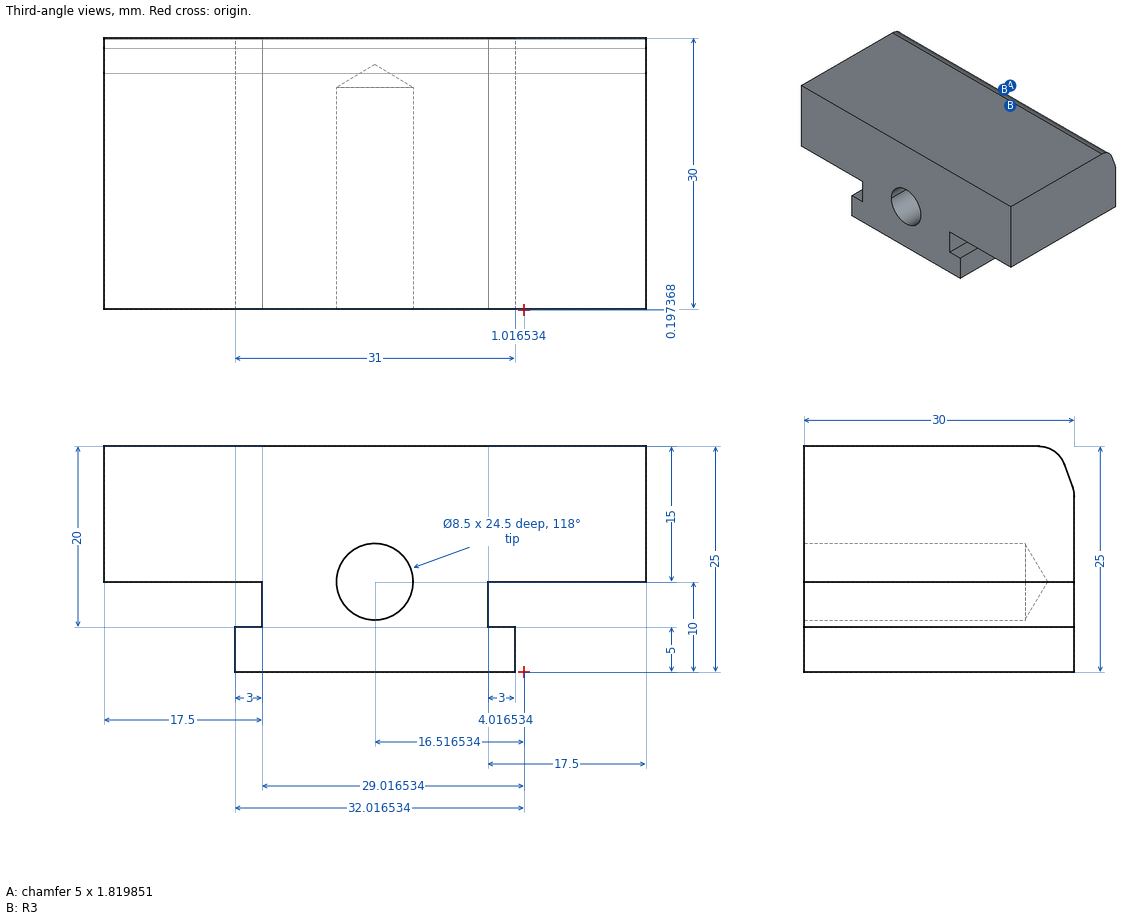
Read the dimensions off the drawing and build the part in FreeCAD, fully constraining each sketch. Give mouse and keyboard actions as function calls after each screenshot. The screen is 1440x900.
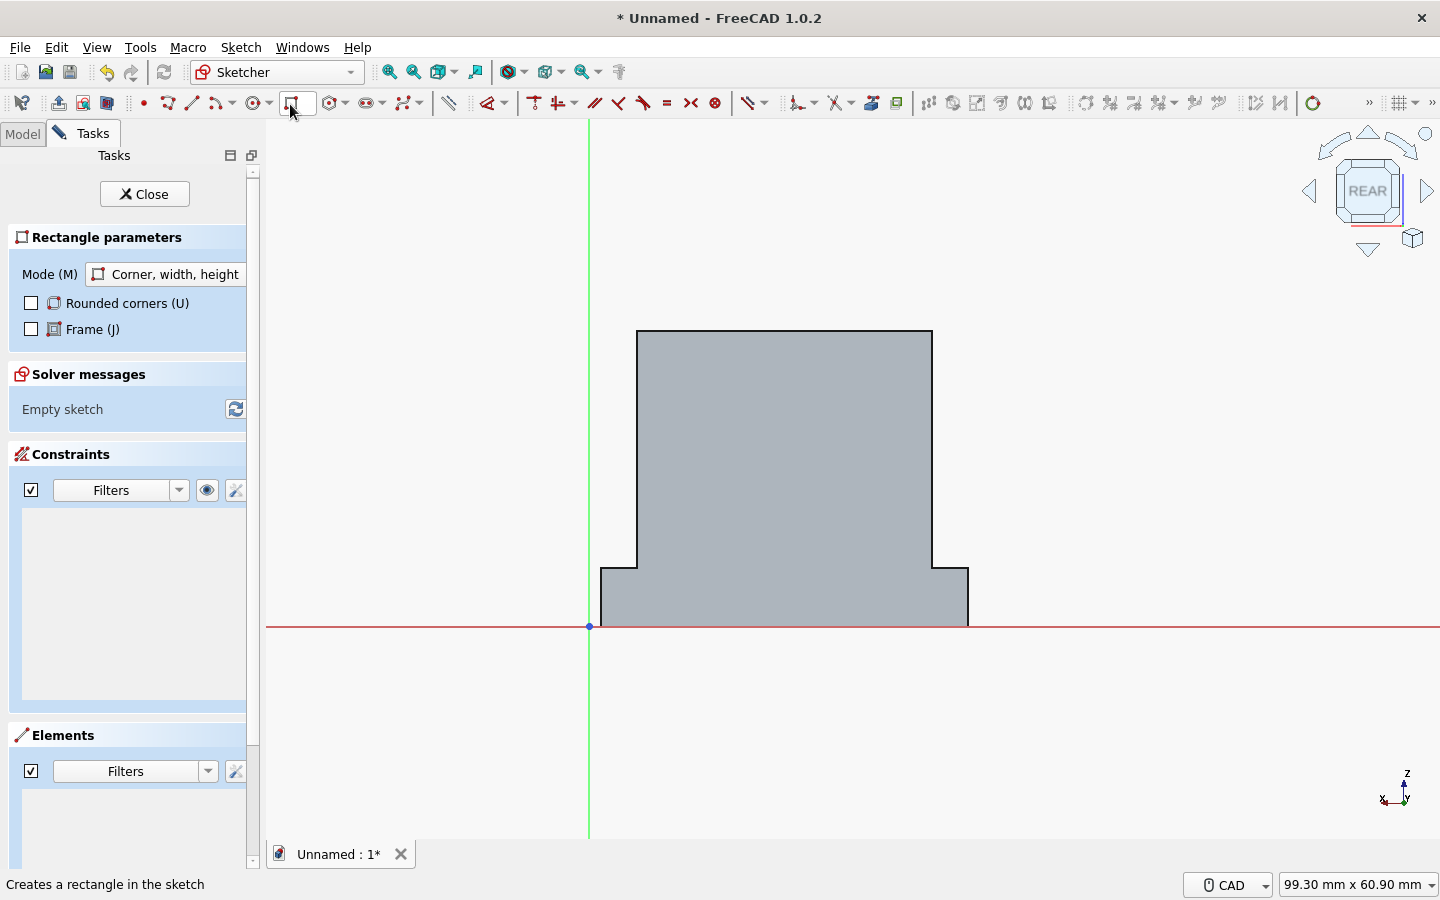
click(430, 331)
move(637, 509)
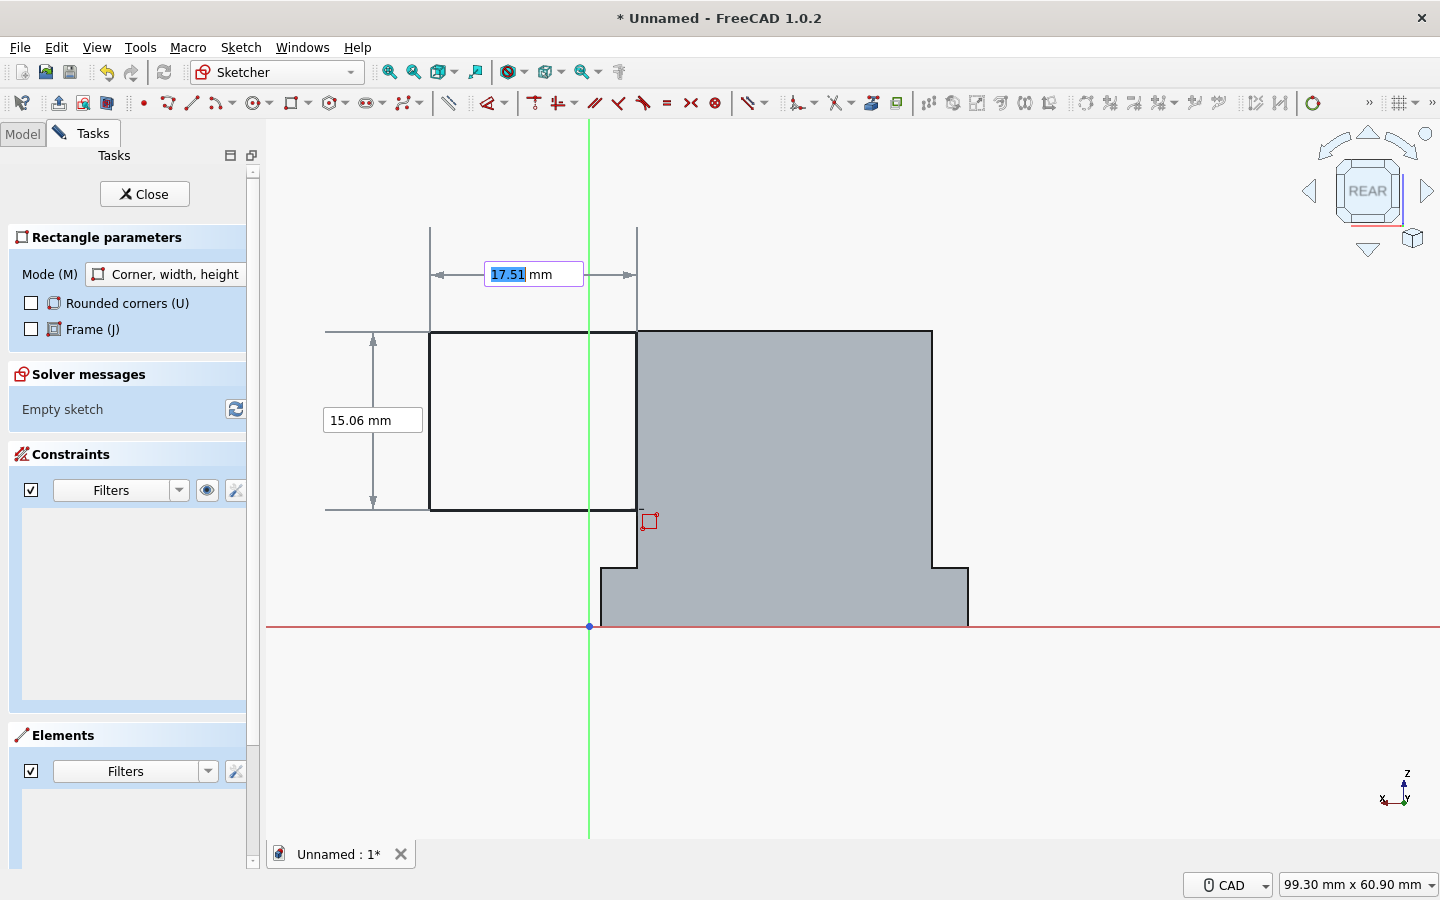
text(17.5)
key(Tab)
text(15)
key(Return)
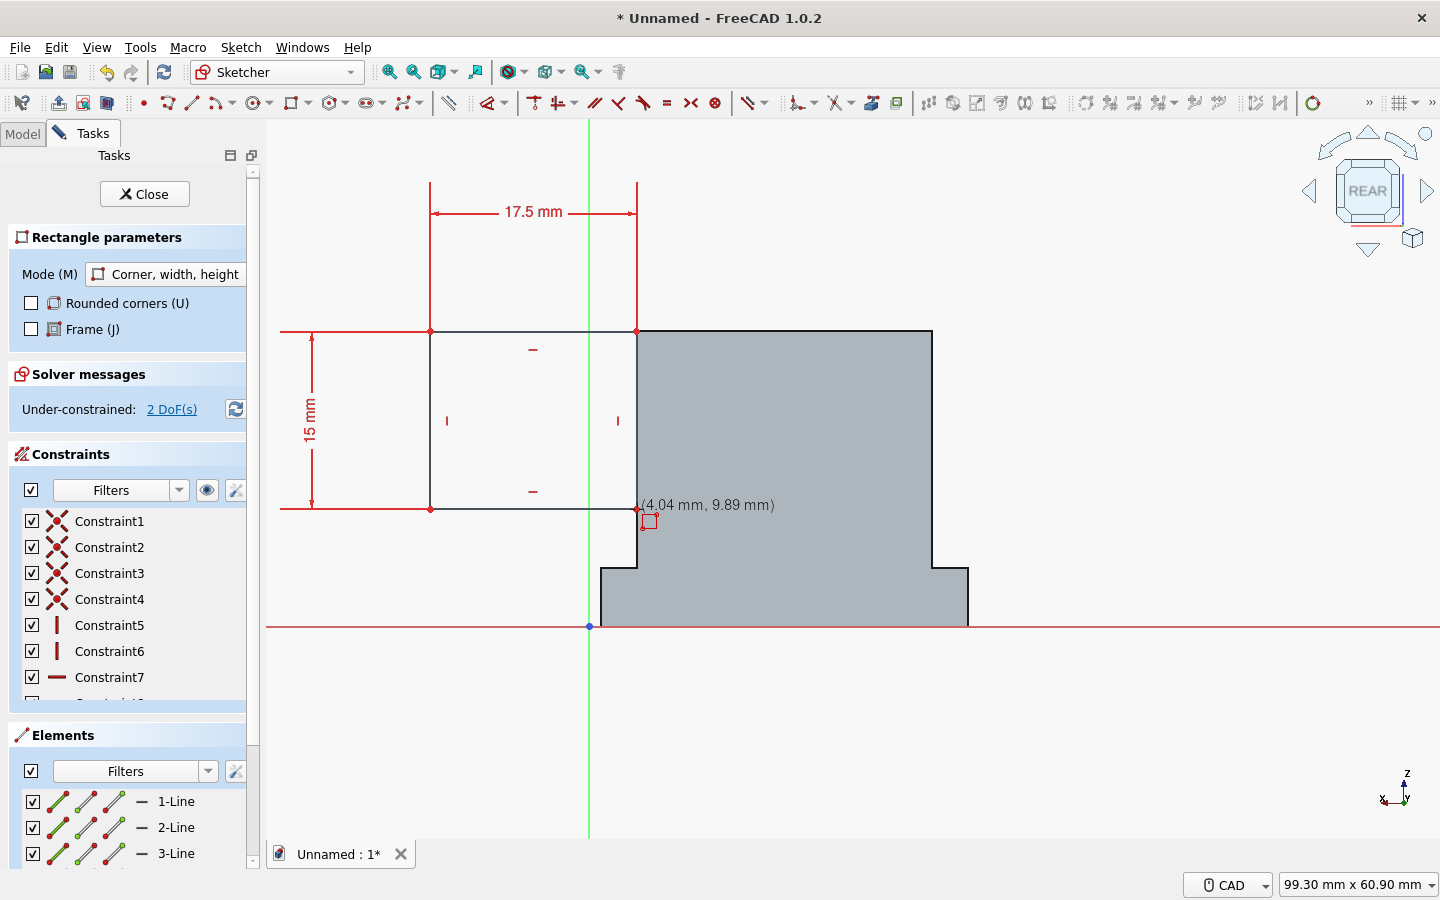
click(932, 331)
move(1139, 509)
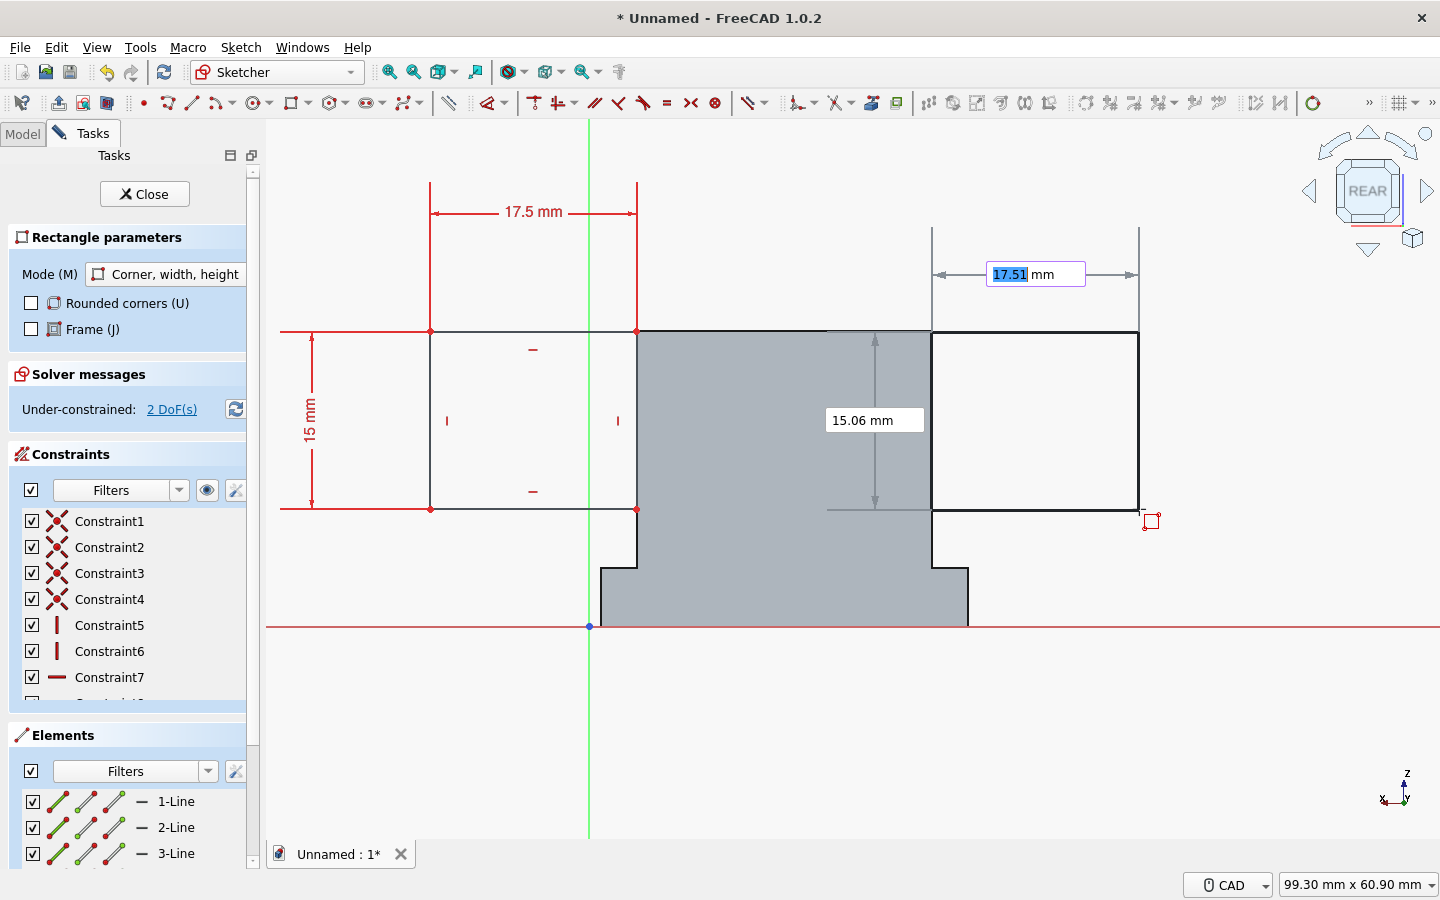
text(17.5)
key(Tab)
text(15)
key(Return)
key(Escape)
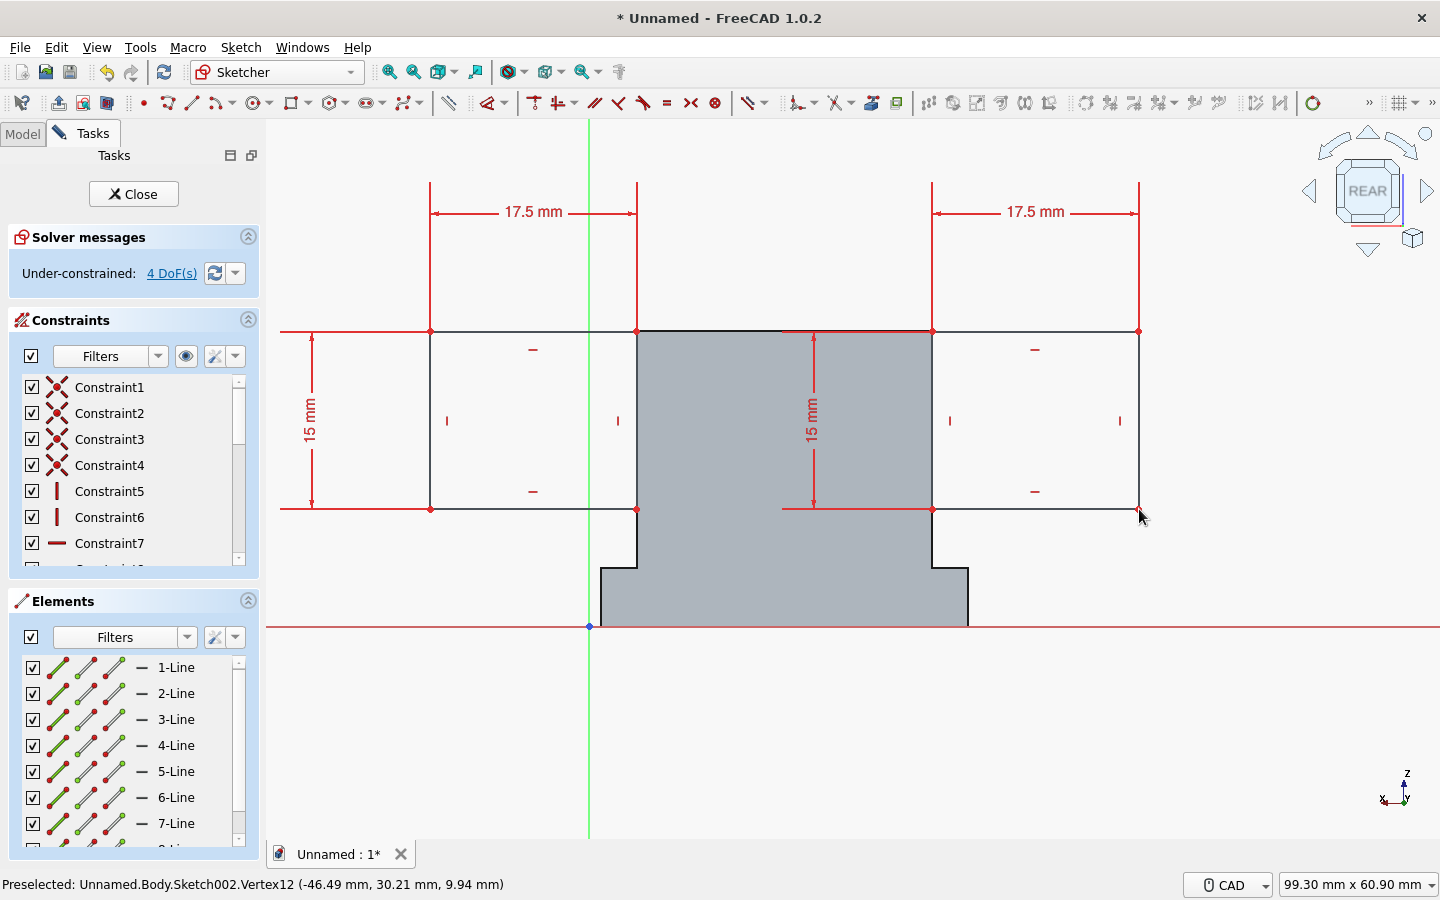
click(488, 104)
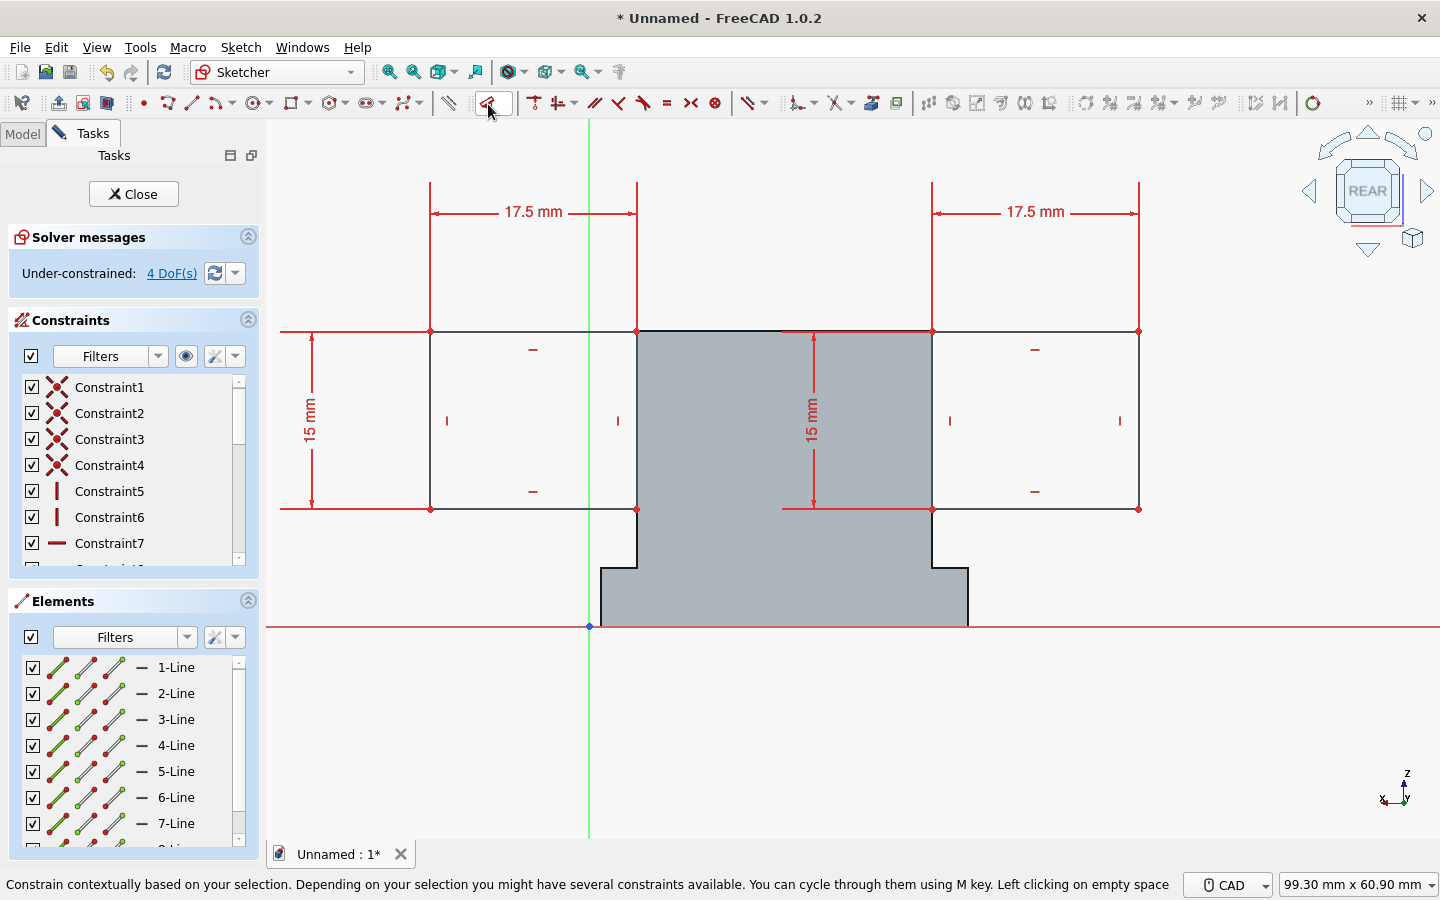
click(430, 332)
click(396, 479)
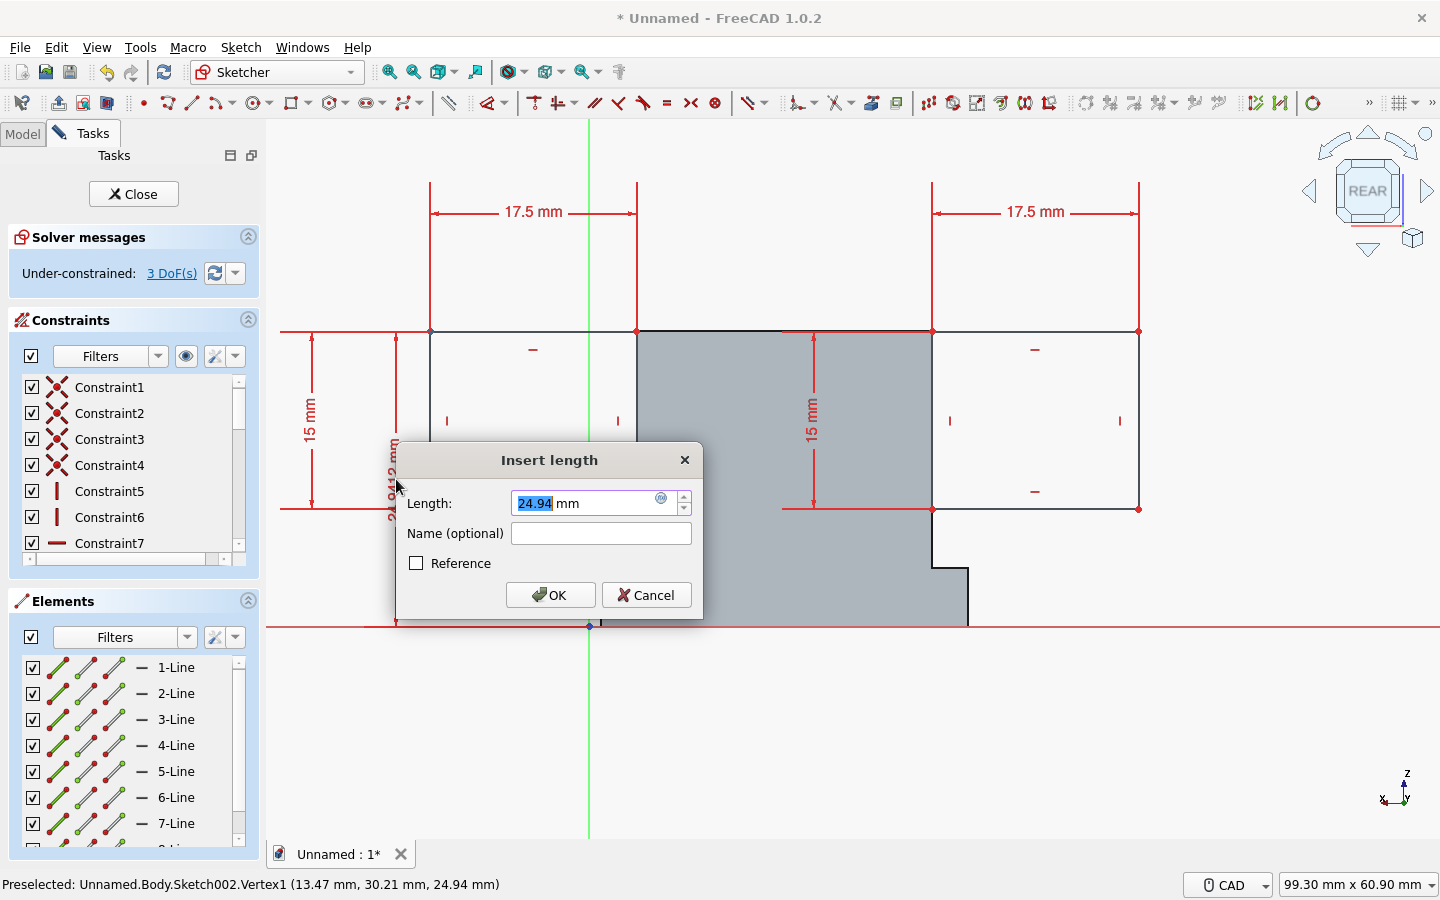
text(25)
key(Return)